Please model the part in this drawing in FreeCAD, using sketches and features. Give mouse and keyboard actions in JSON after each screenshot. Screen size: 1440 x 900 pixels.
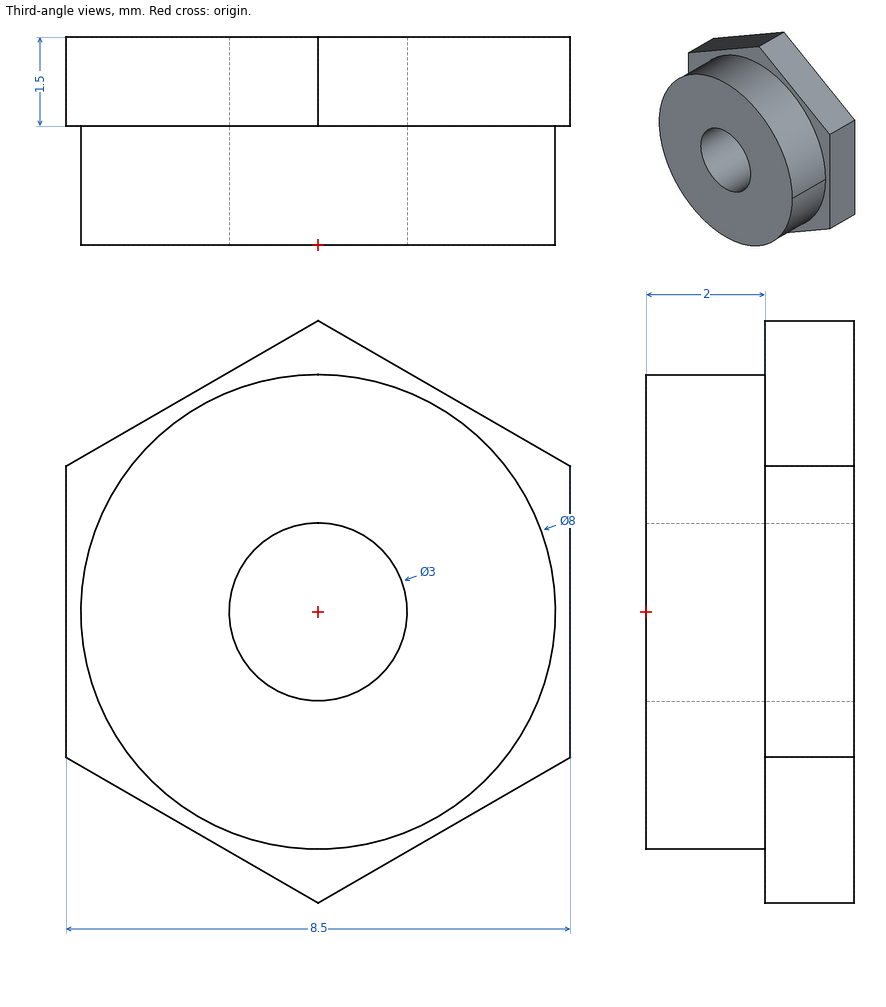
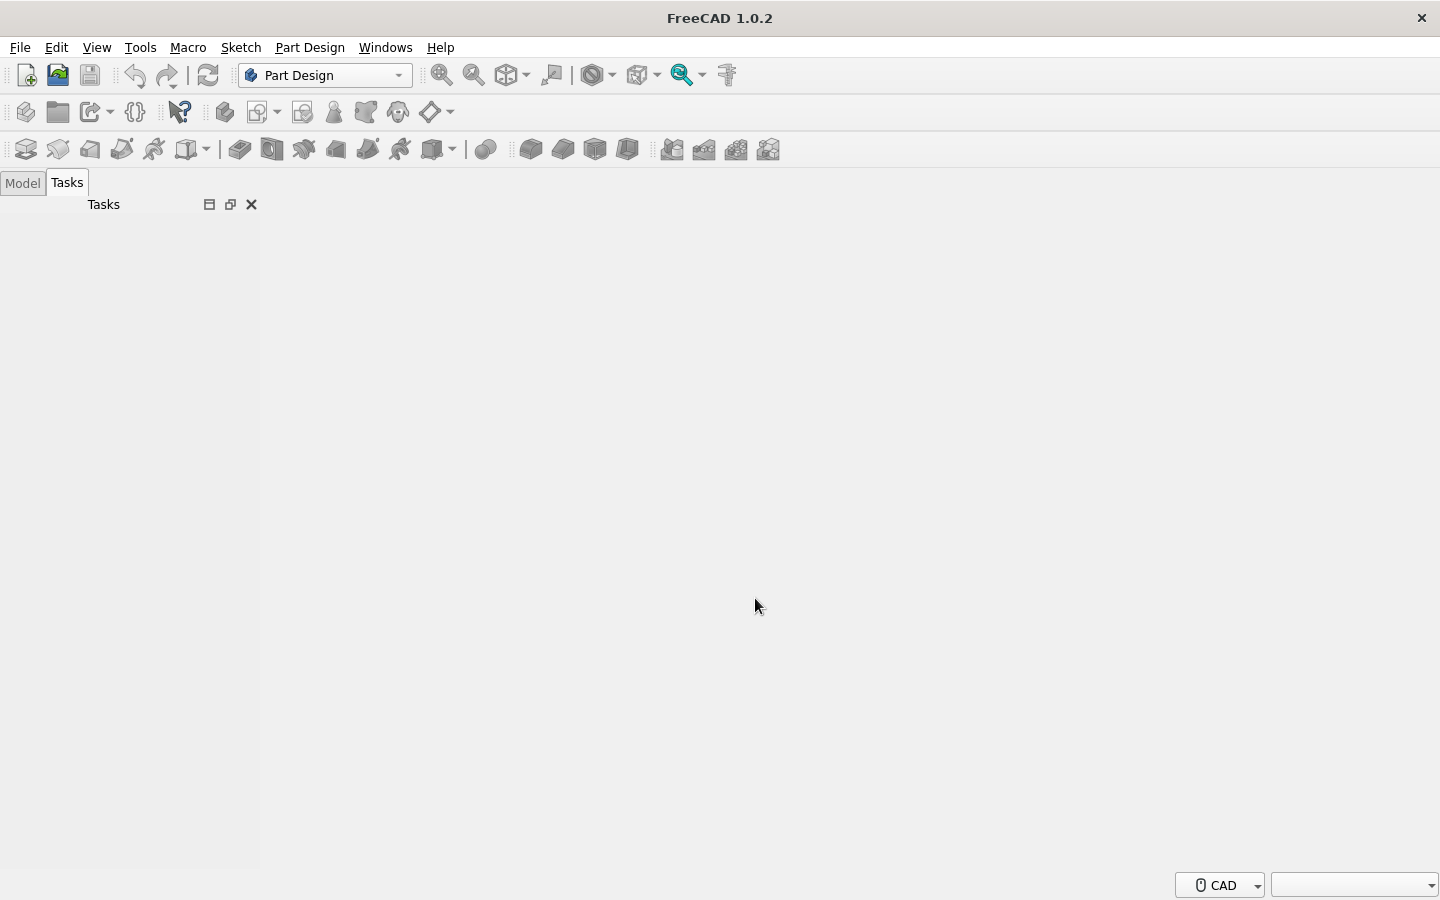
{"action": "left_click", "coordinate": [26, 76]}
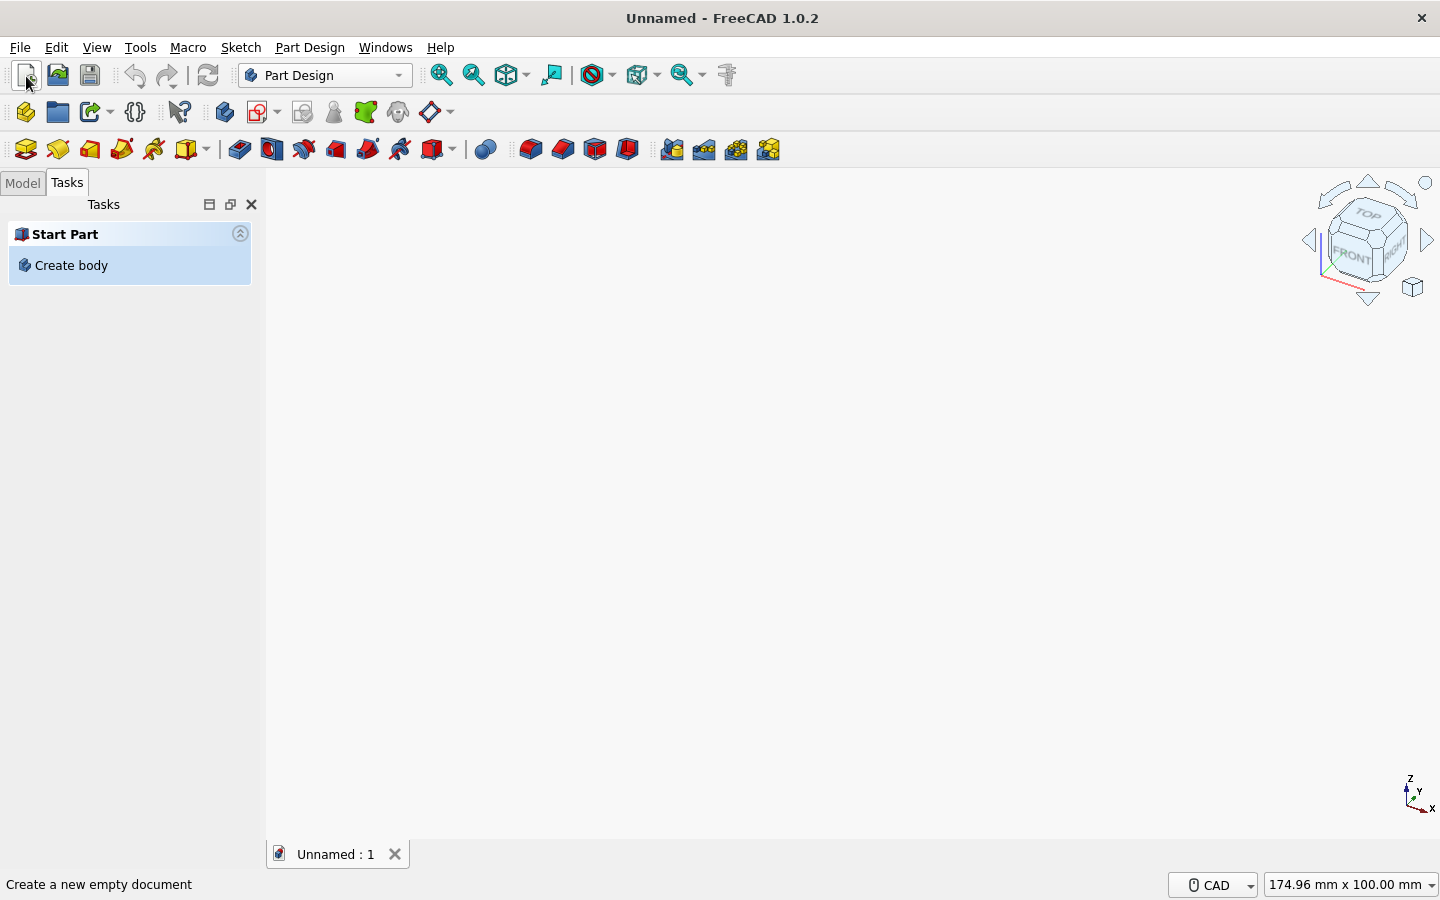
{"action": "left_click", "coordinate": [258, 112]}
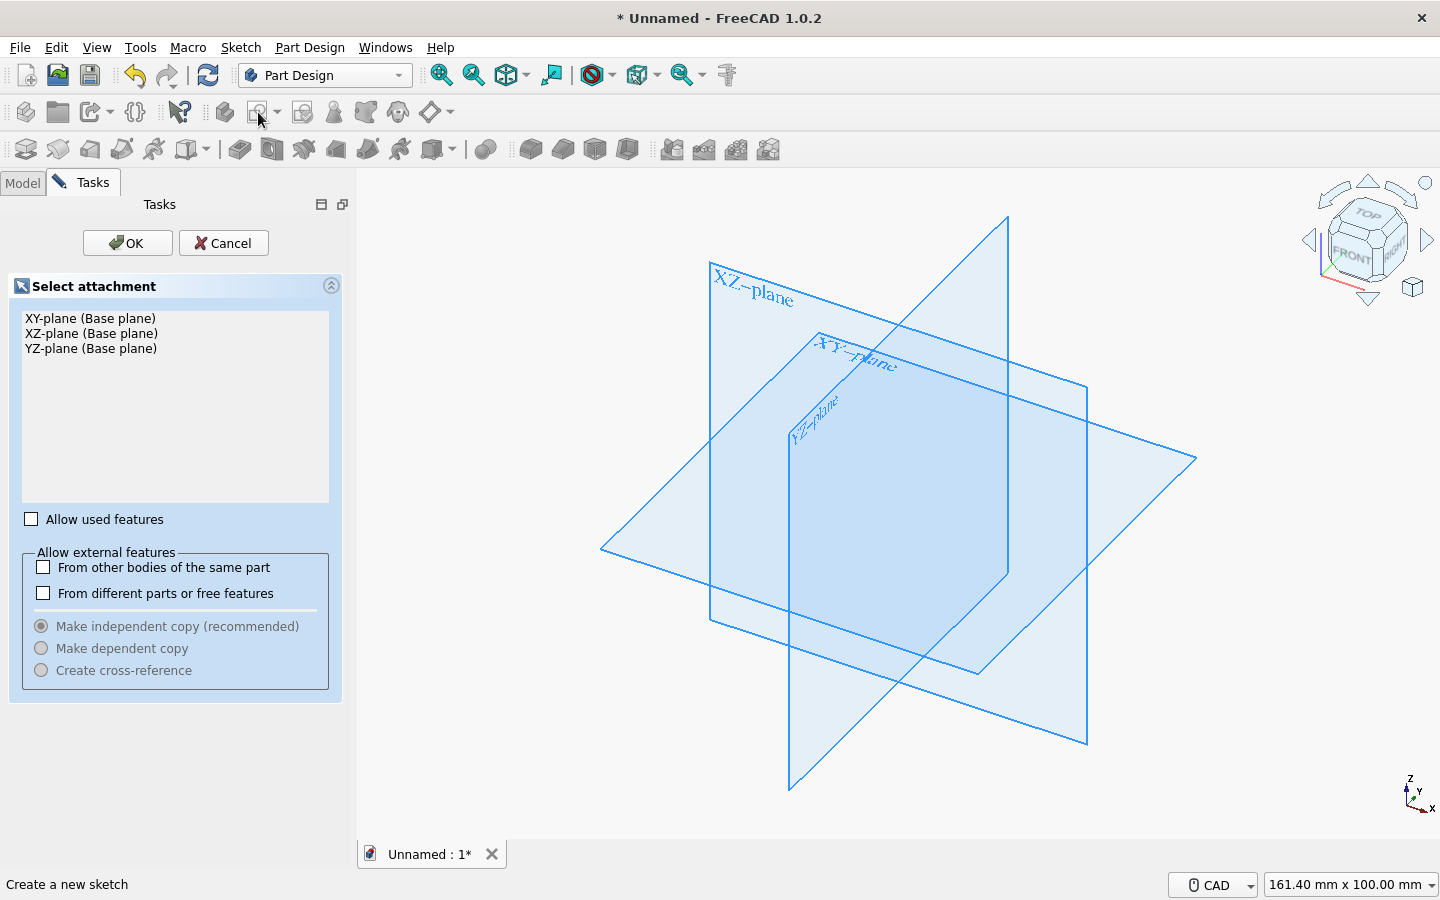
{"action": "left_click", "coordinate": [82, 334]}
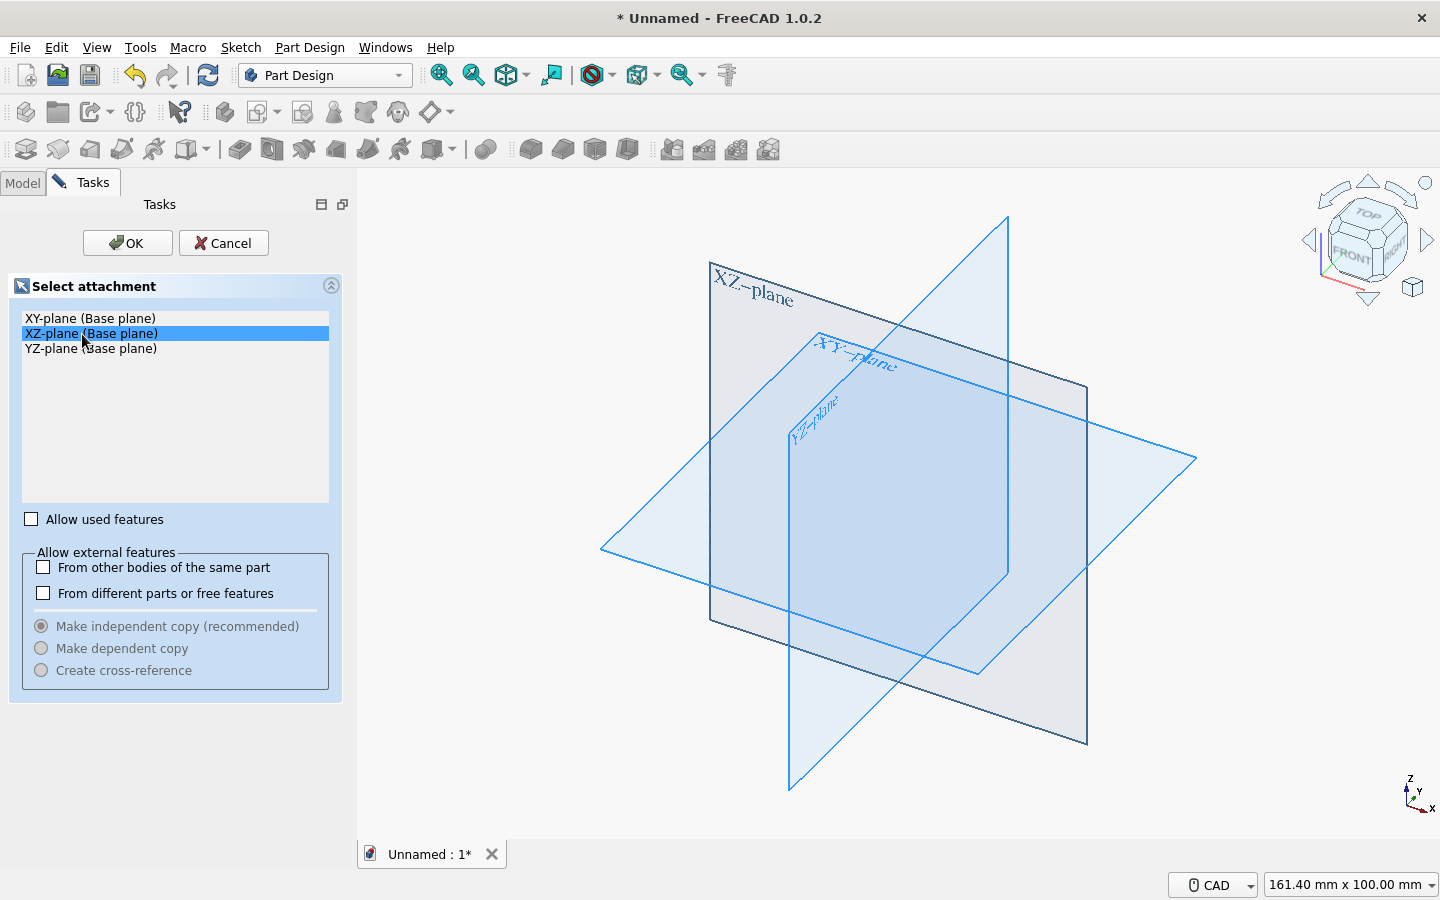
{"action": "left_click", "coordinate": [128, 243]}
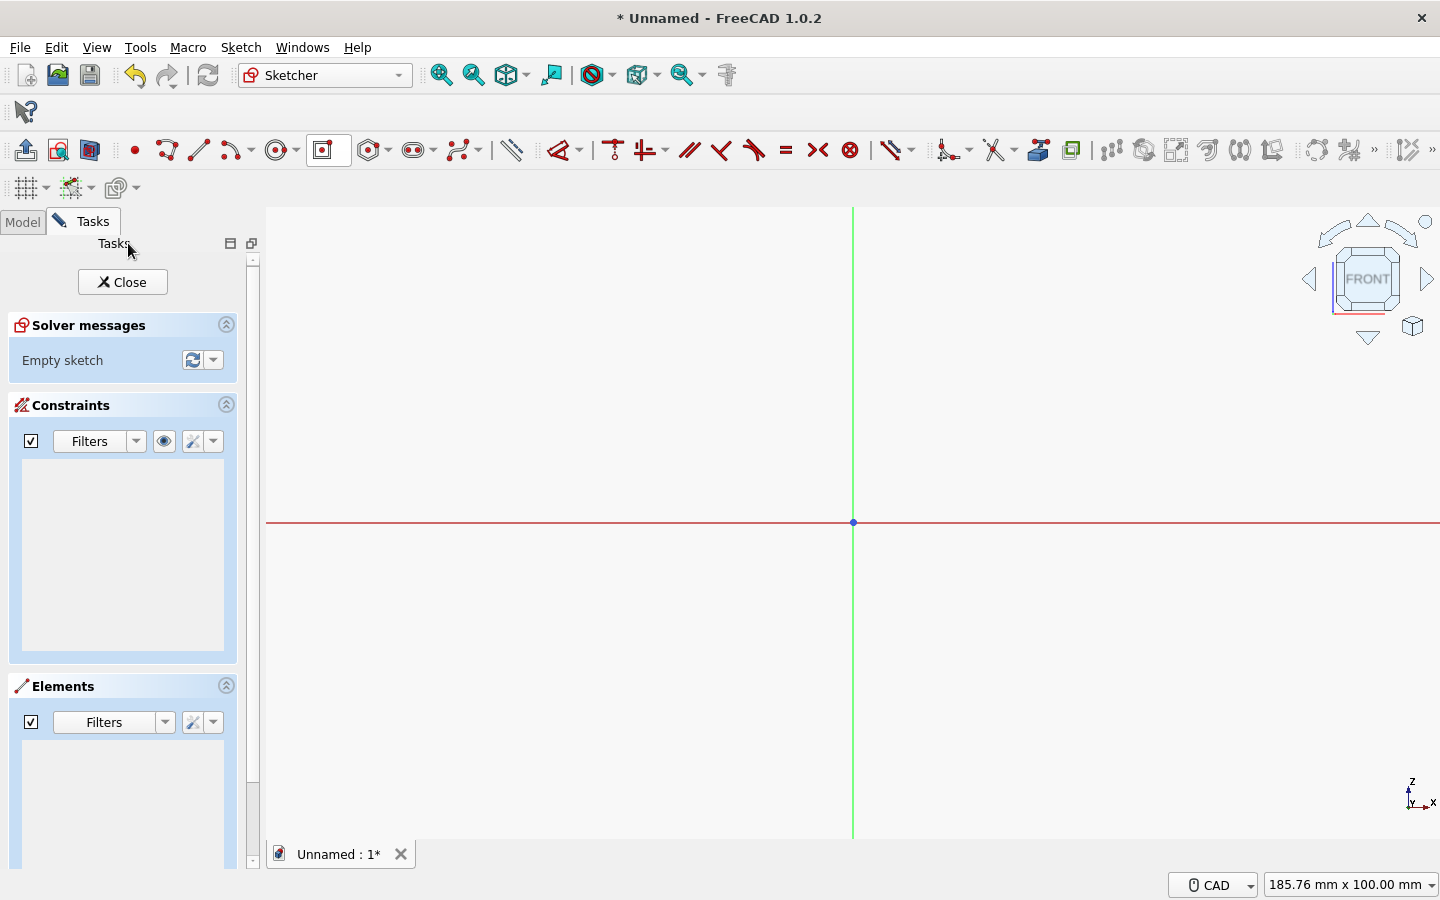
{"action": "scroll", "coordinate": [864, 523], "scroll_direction": "up", "scroll_amount": 10}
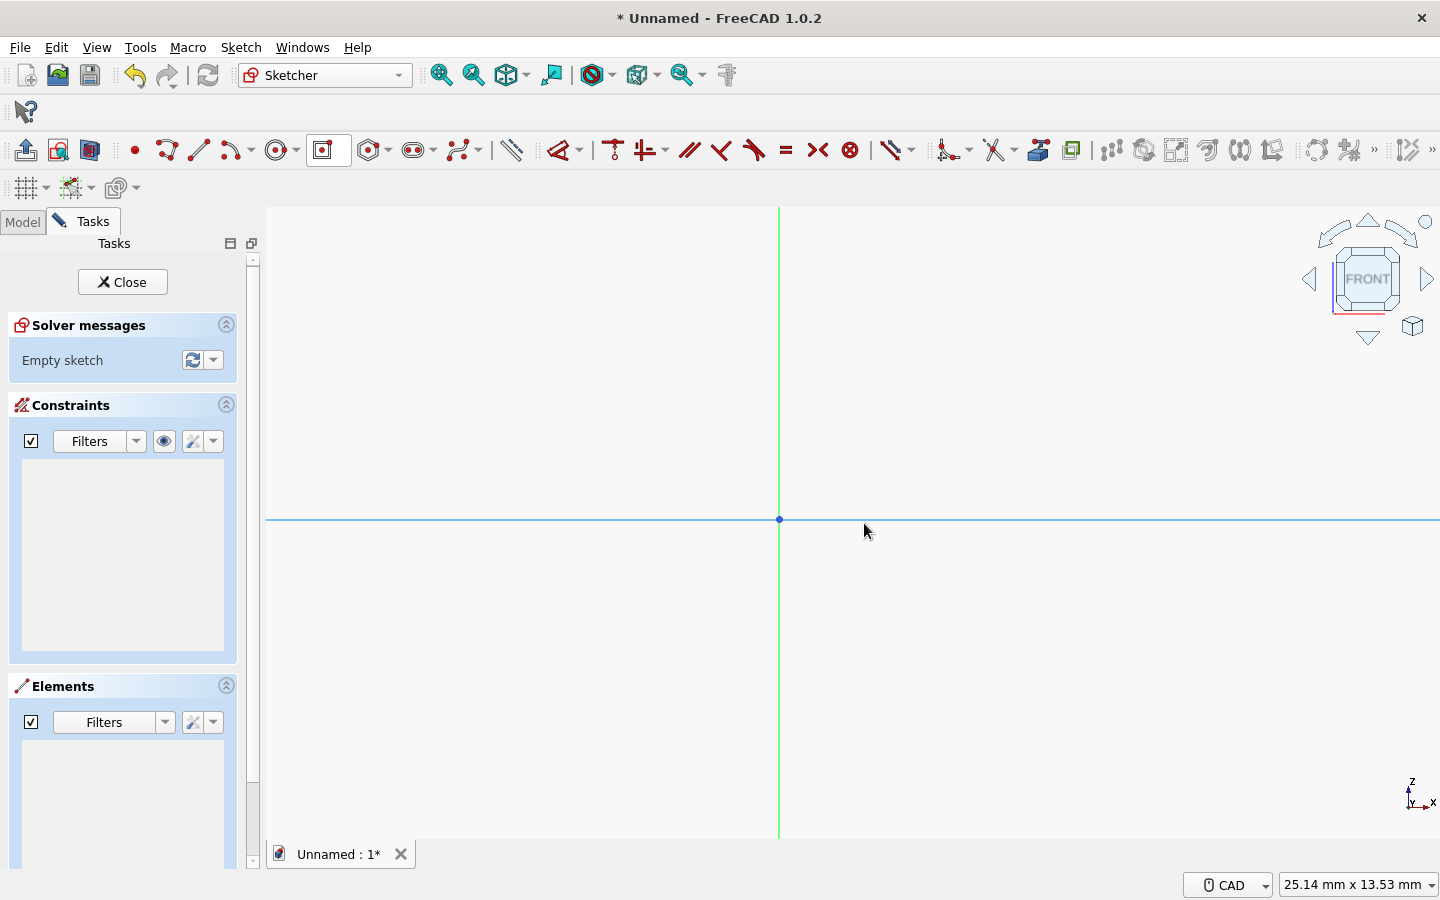
{"action": "key", "text": "g c"}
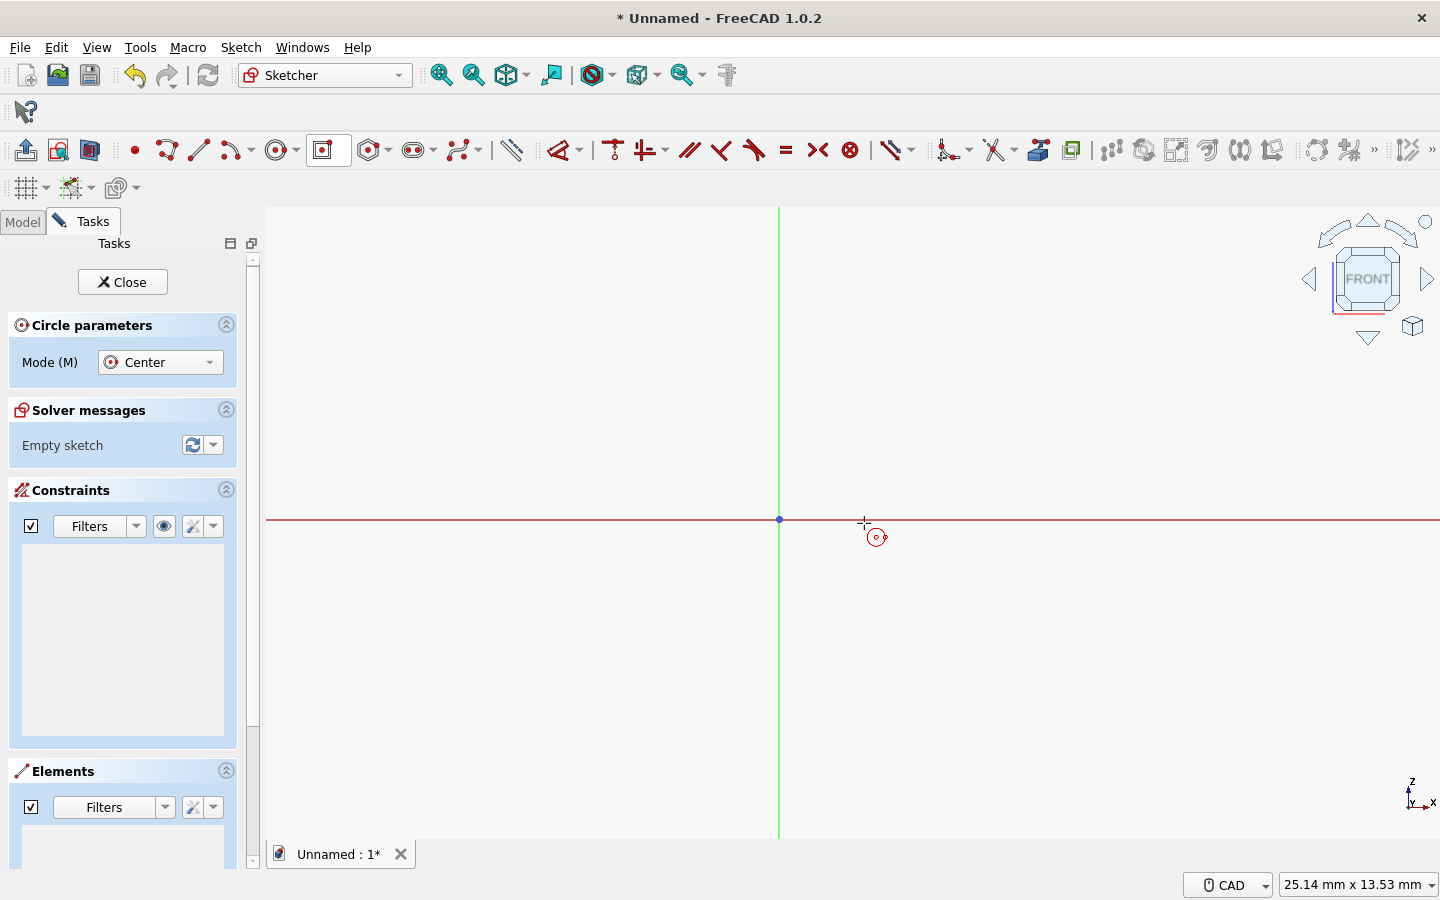
{"action": "left_click", "coordinate": [779, 520]}
{"action": "mouse_move", "coordinate": [912, 388]}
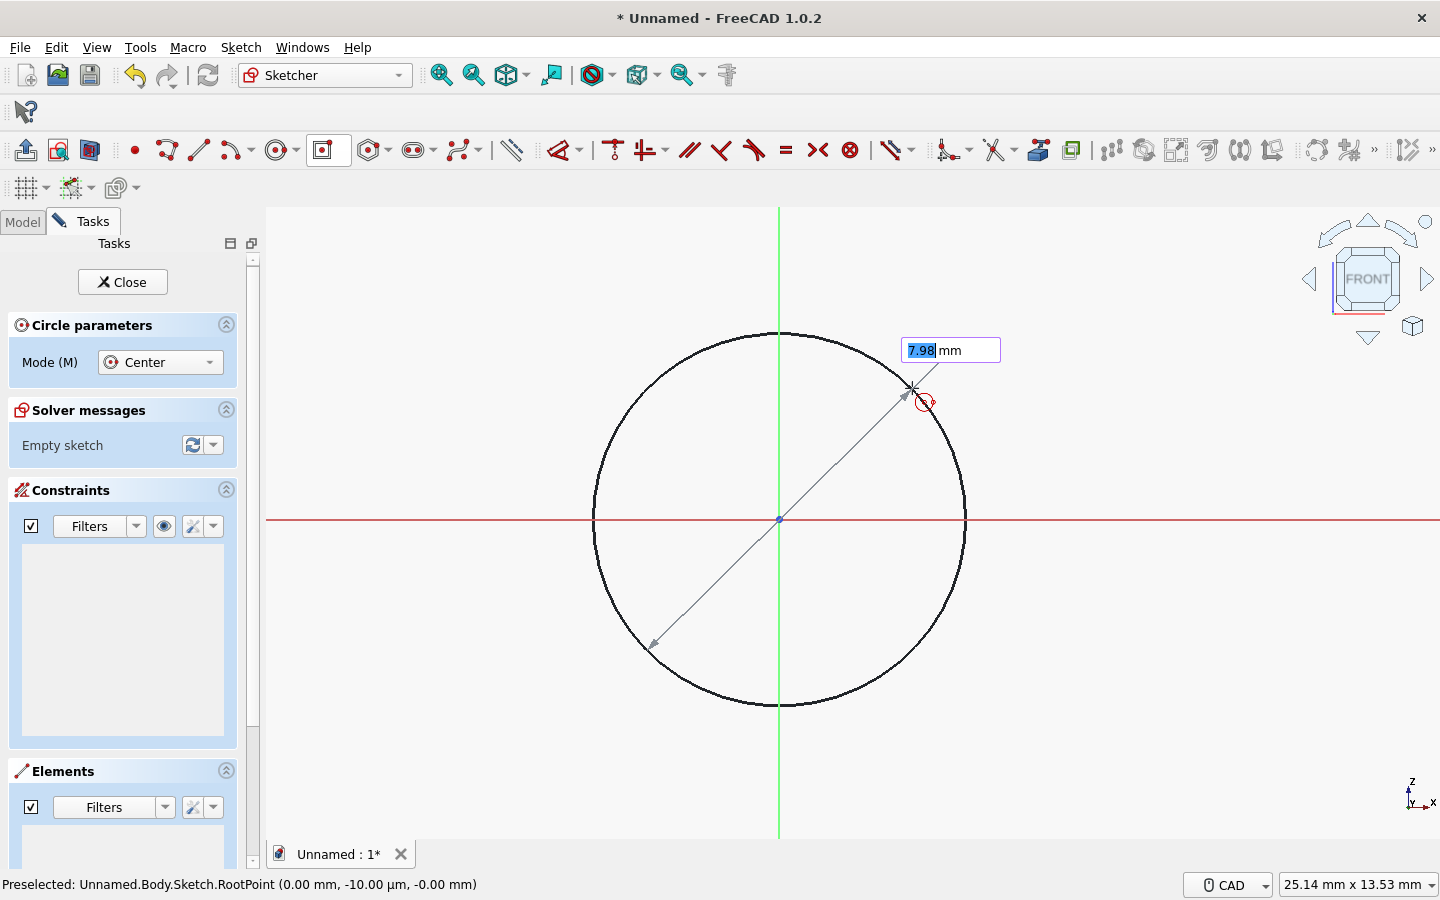
{"action": "type", "text": "8"}
{"action": "key", "text": "Return"}
{"action": "key", "text": "Escape"}